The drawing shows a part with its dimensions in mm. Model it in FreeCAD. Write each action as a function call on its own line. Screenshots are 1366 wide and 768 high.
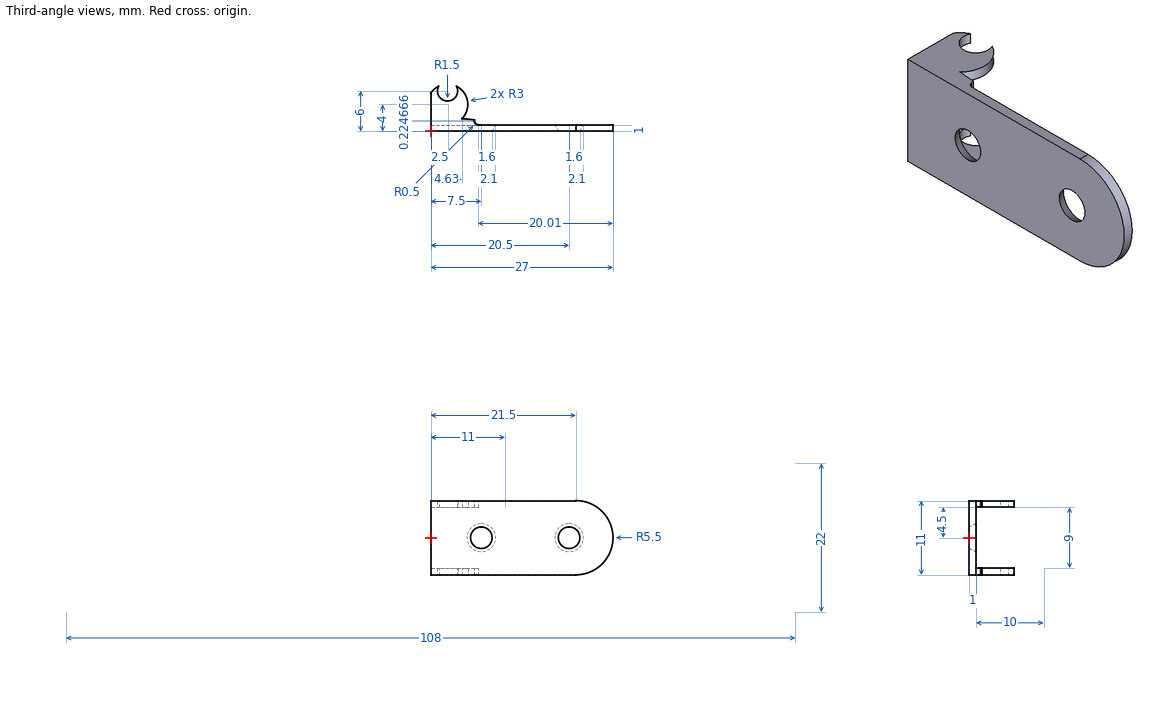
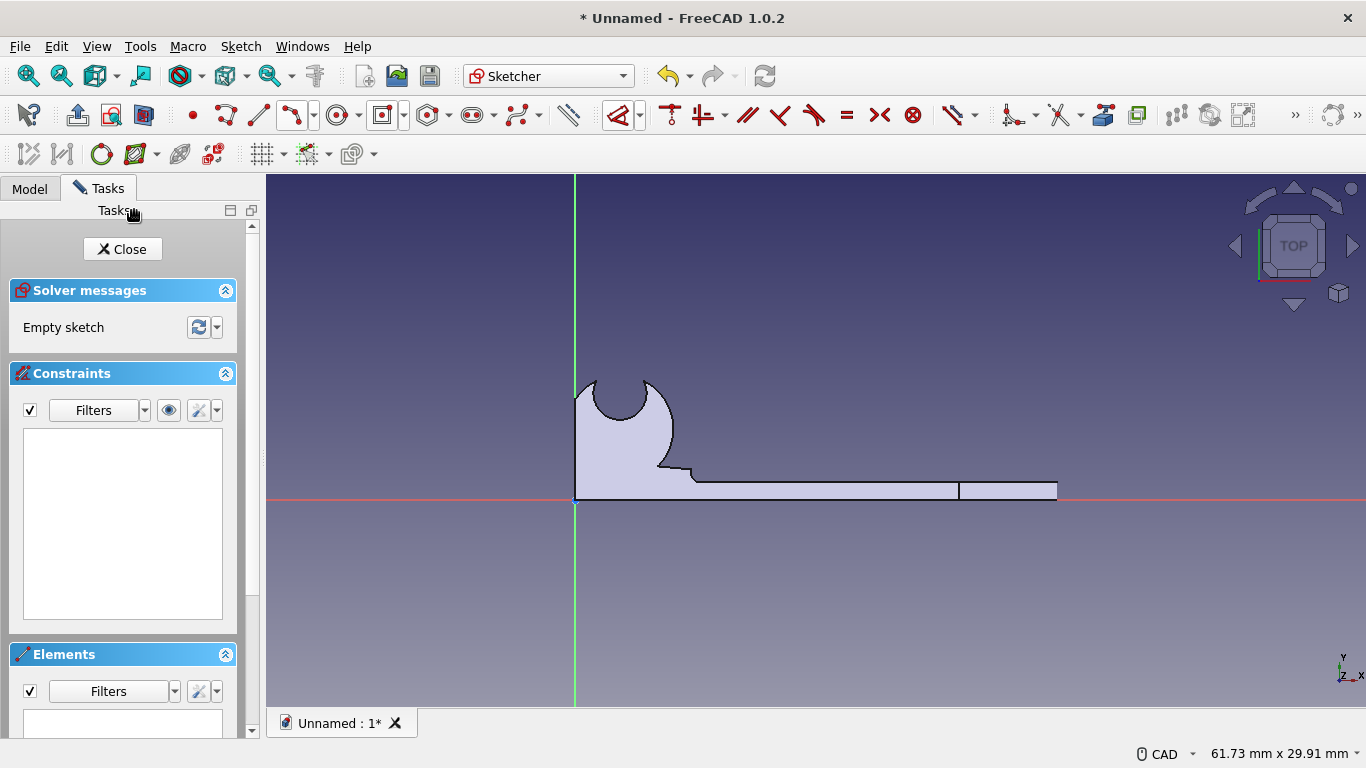
key(q)
key(s)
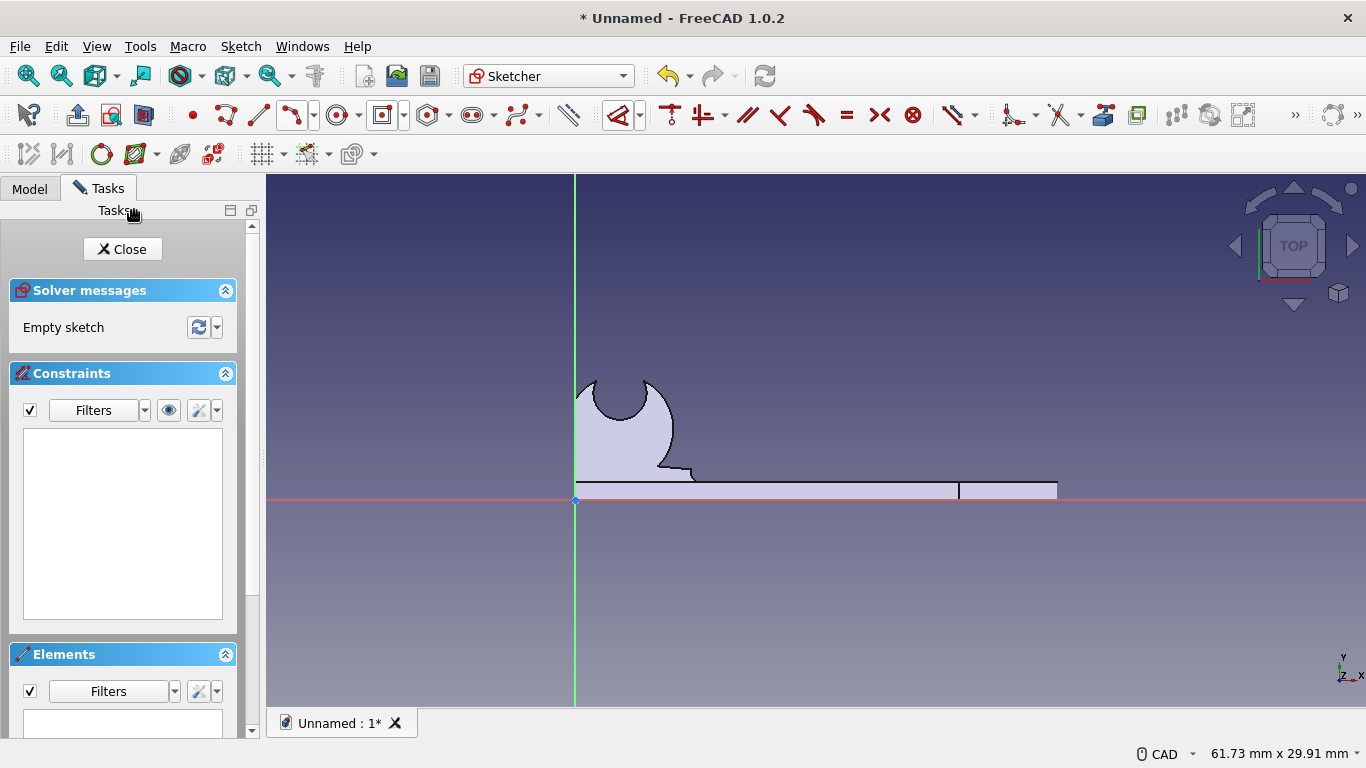
scroll(726, 491, up, 13)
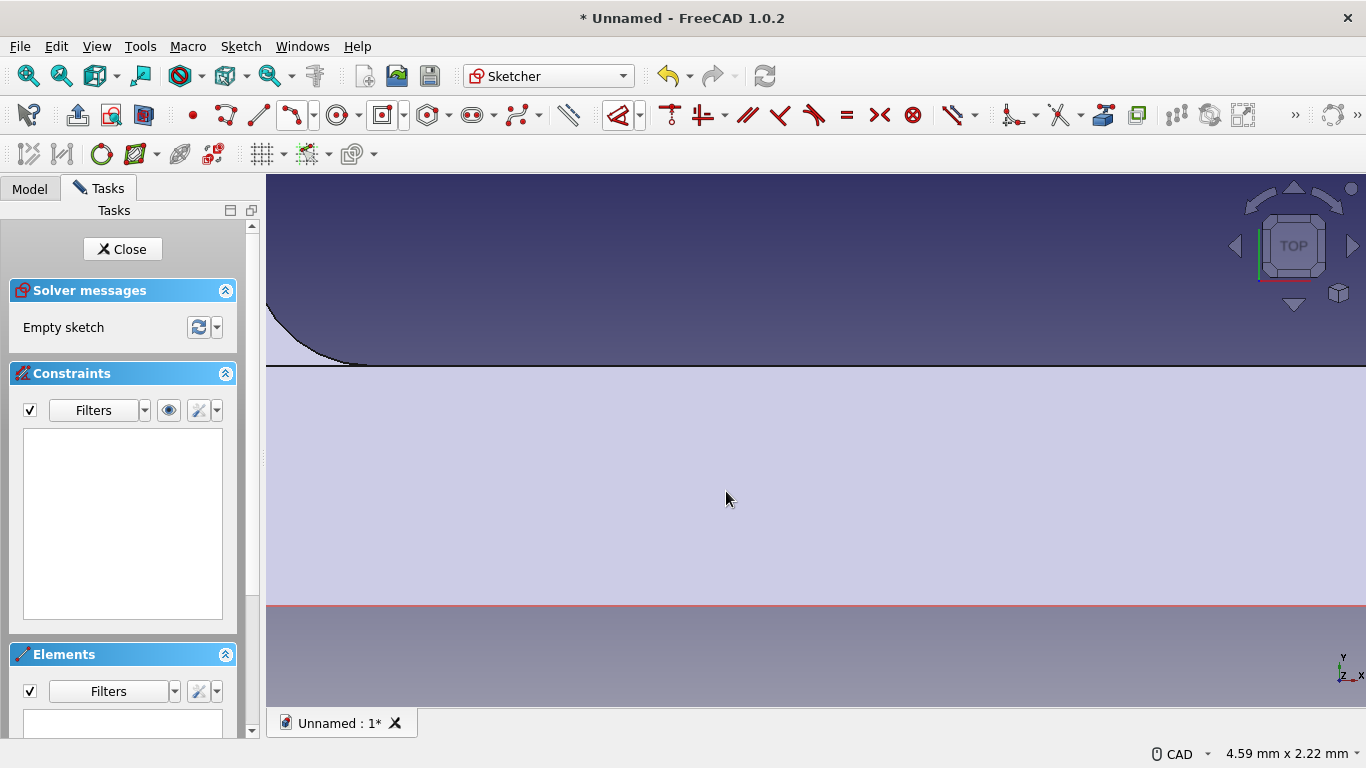
key(g)
key(m)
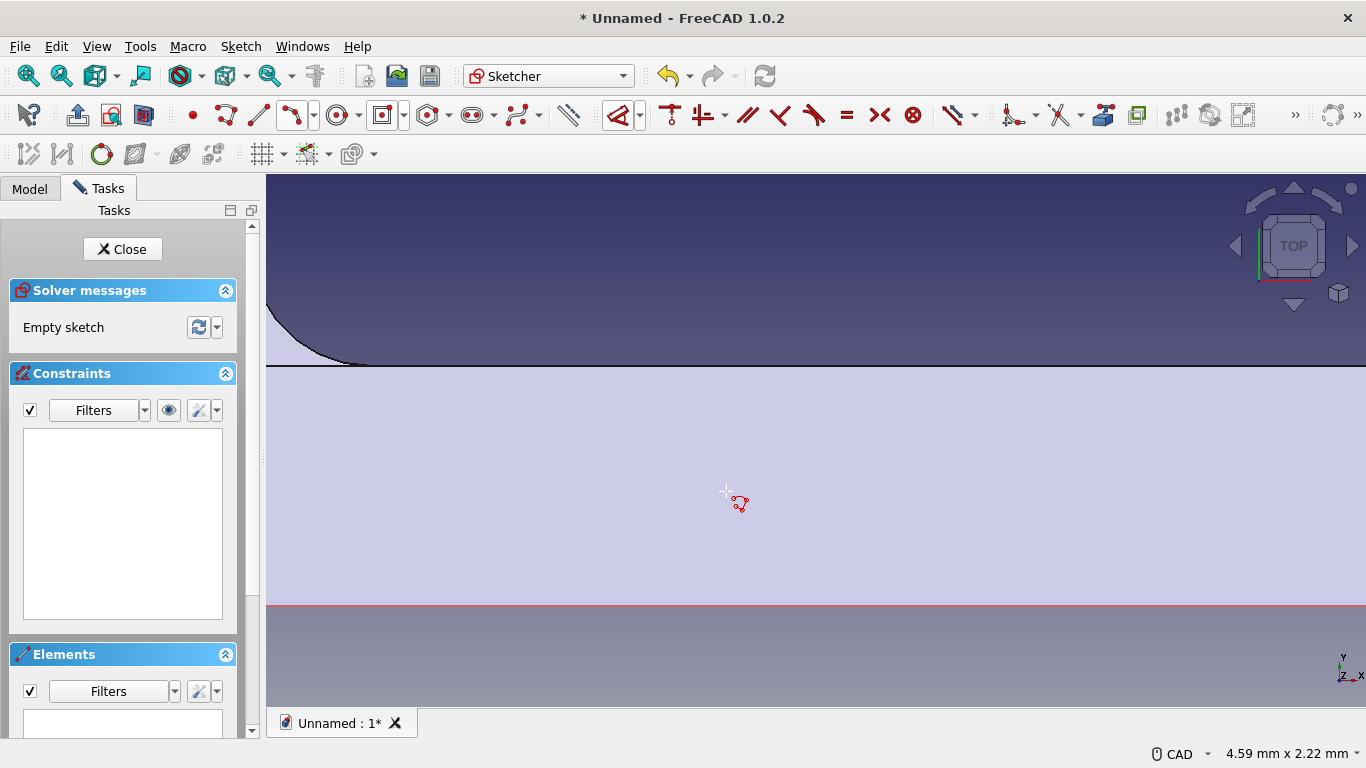
click(493, 606)
click(877, 597)
click(997, 366)
click(493, 366)
click(493, 606)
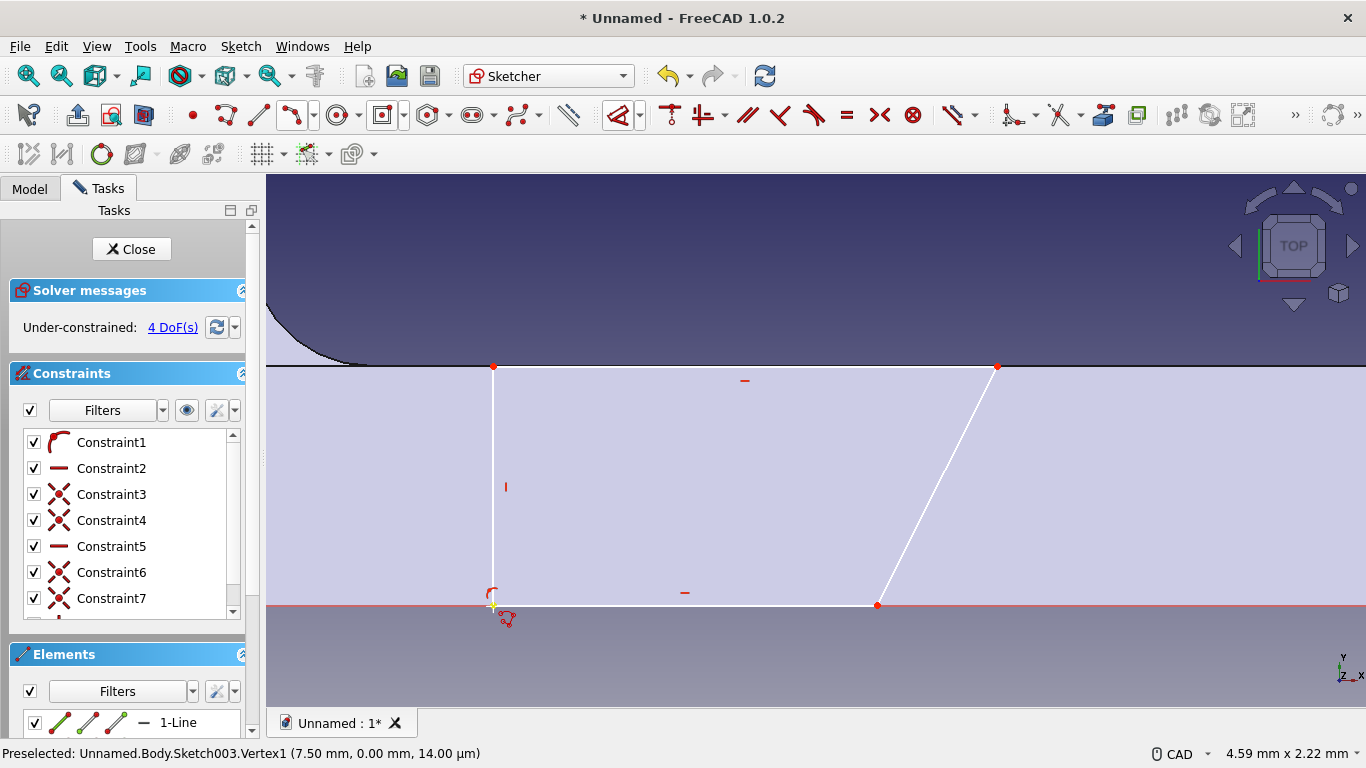
key(g)
key(l)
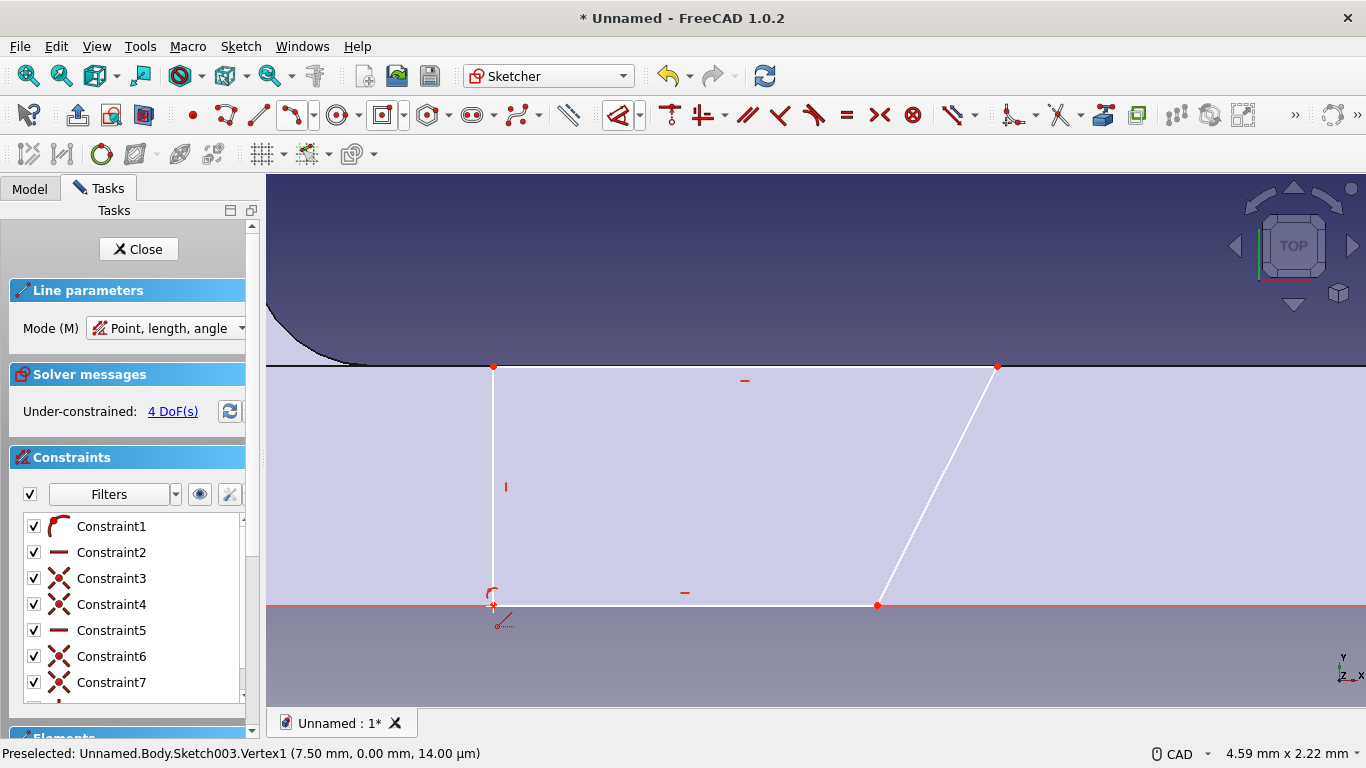
click(493, 342)
click(493, 270)
key(Escape)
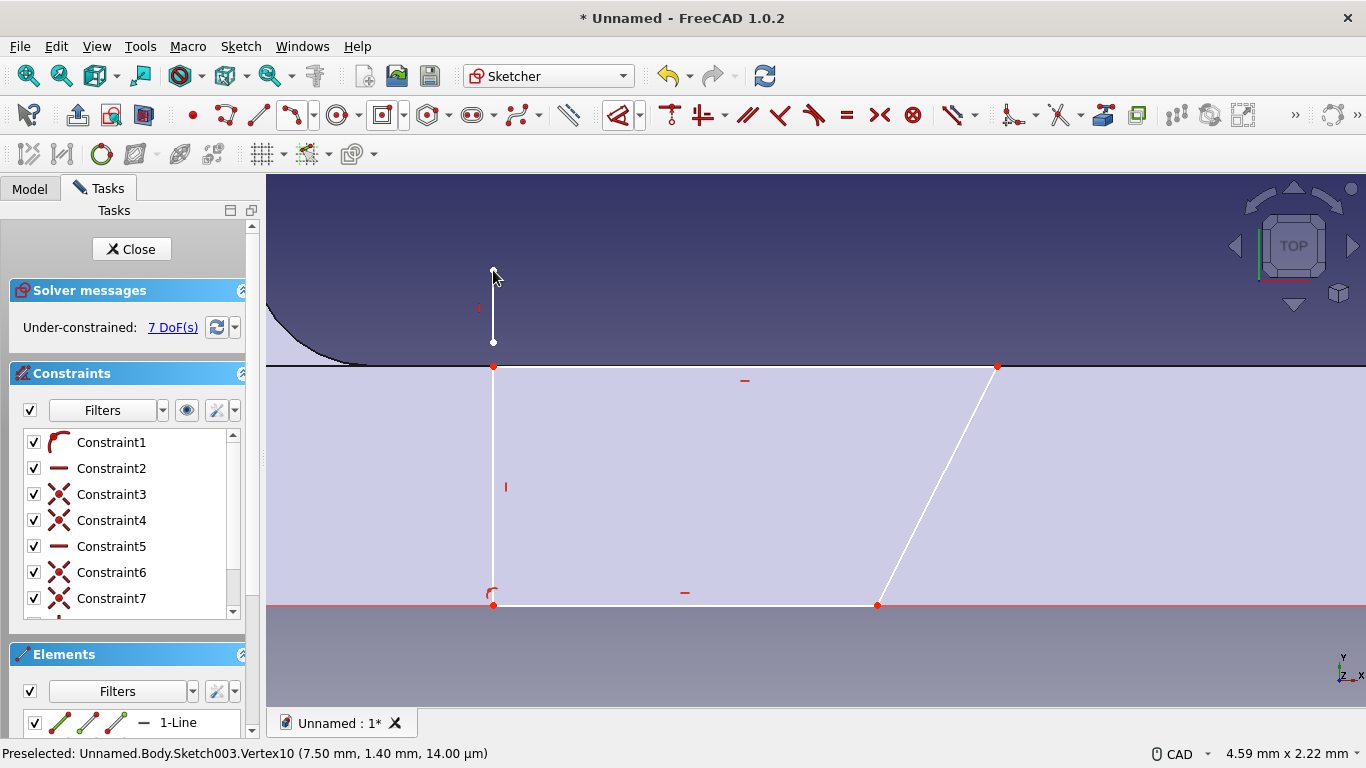
click(493, 321)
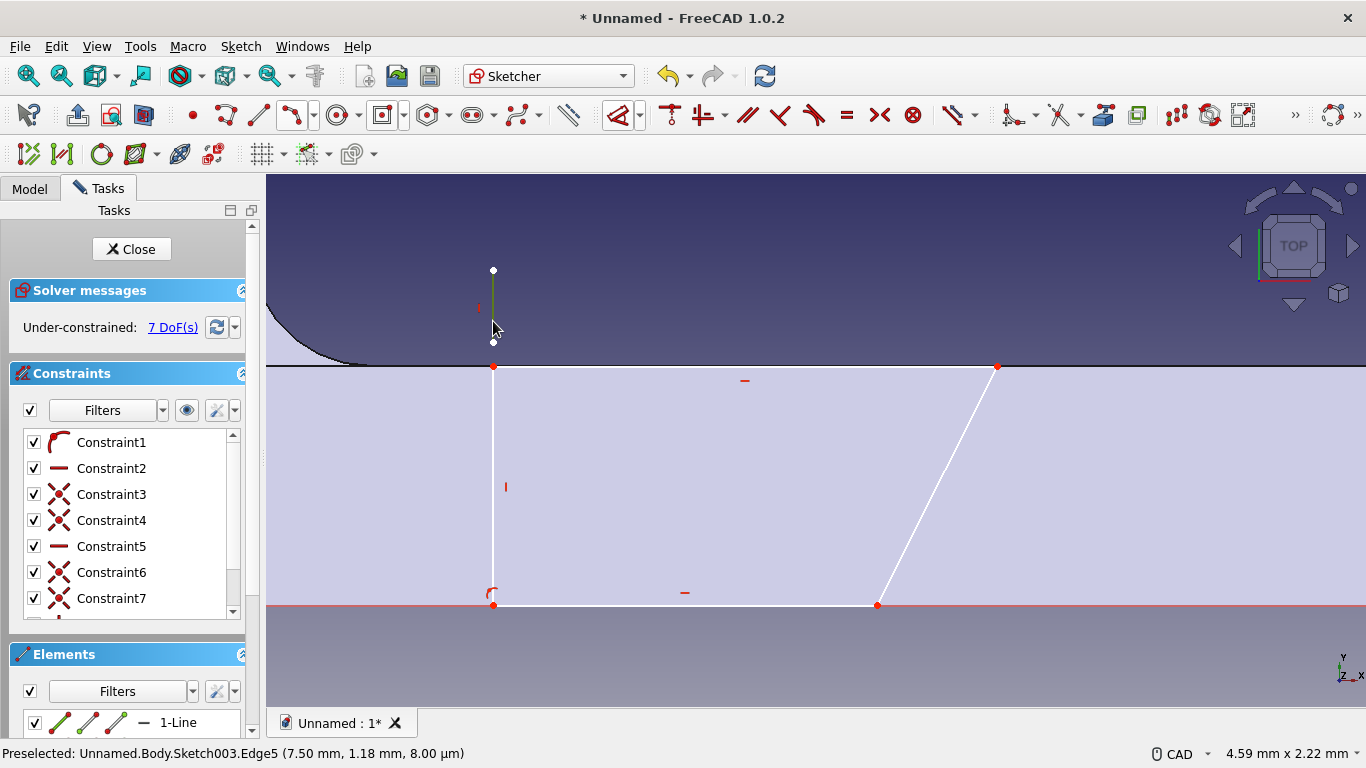
click(569, 116)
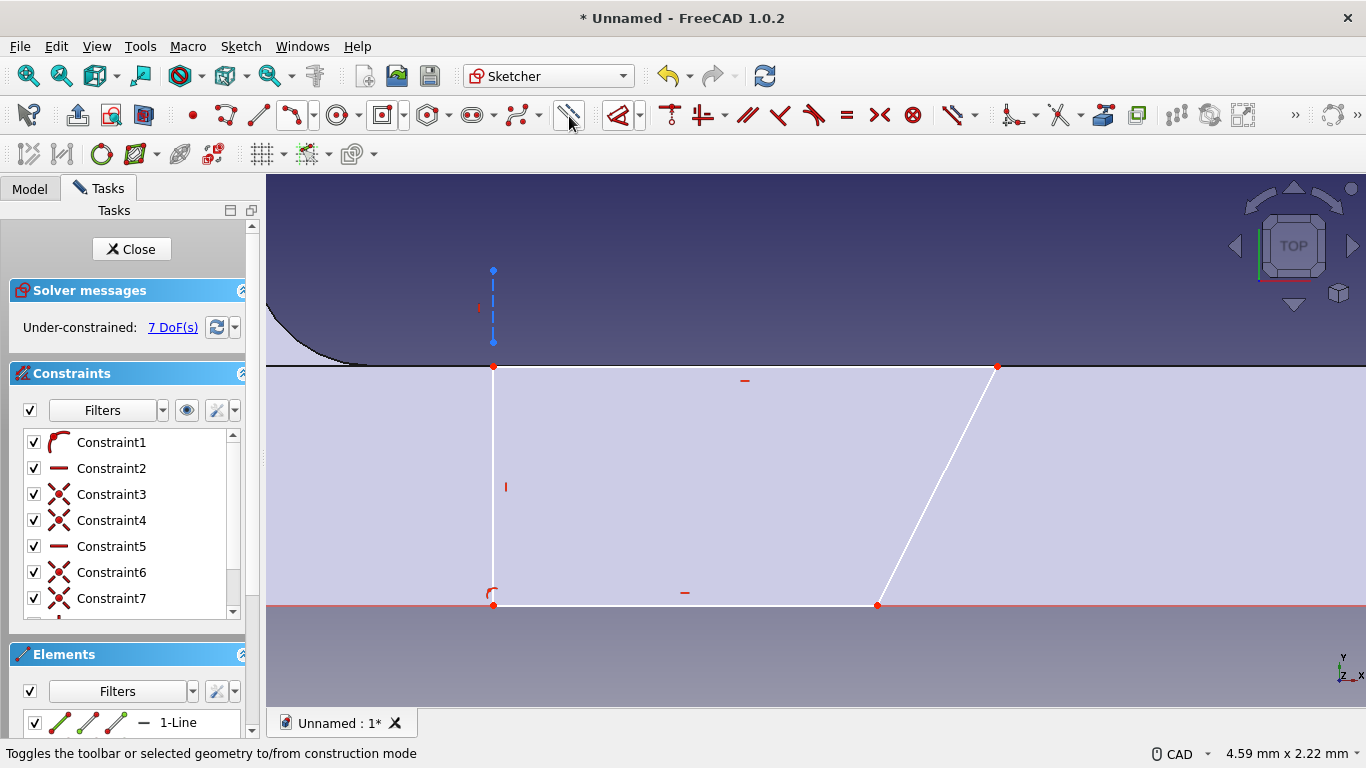
click(493, 439)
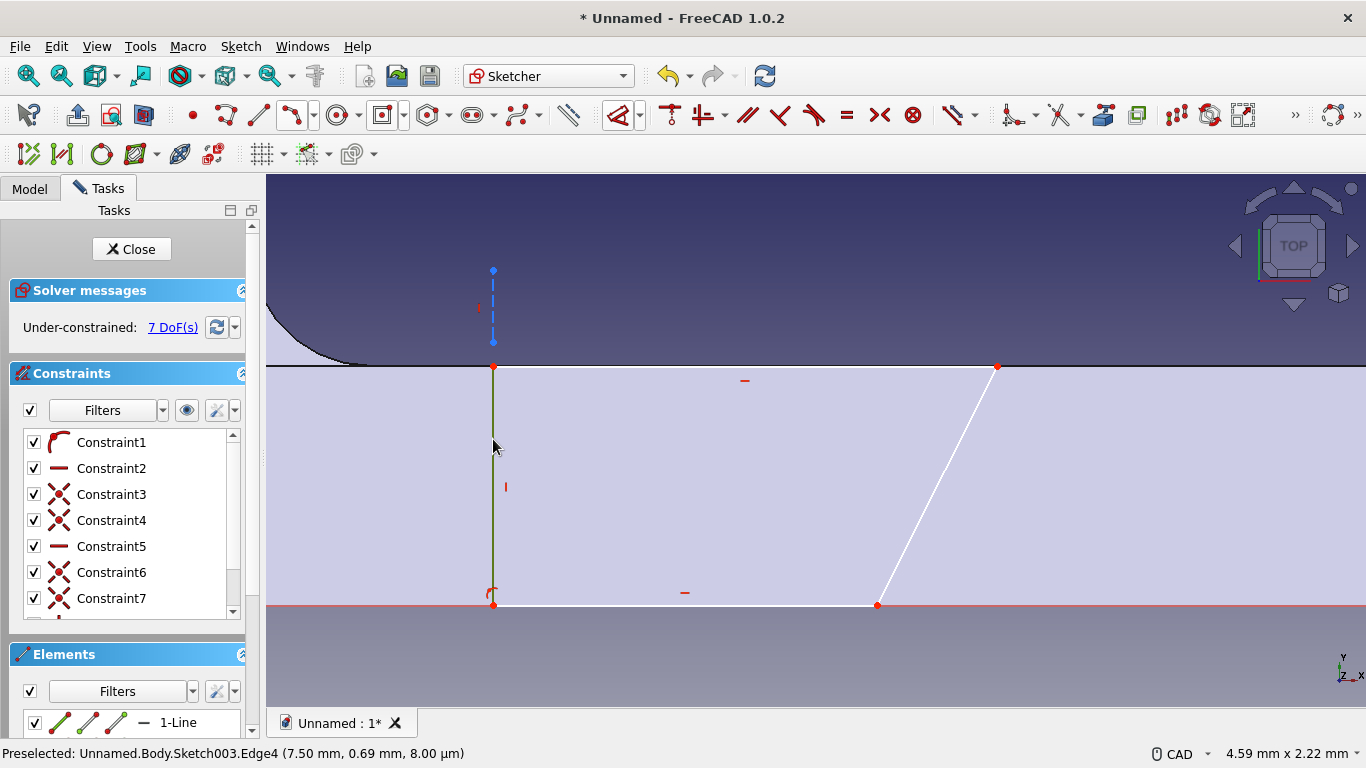
key(i)